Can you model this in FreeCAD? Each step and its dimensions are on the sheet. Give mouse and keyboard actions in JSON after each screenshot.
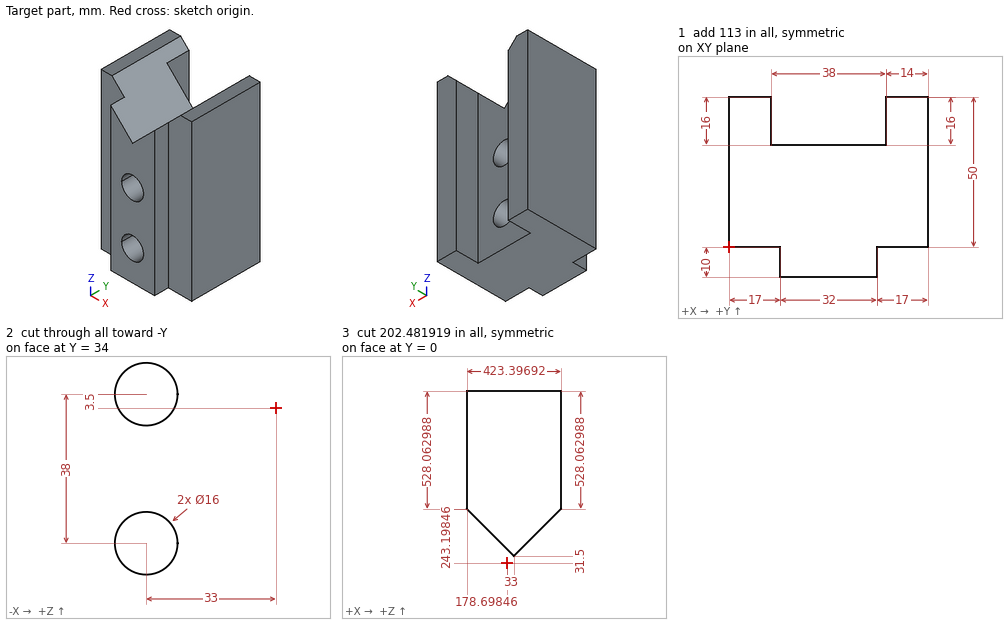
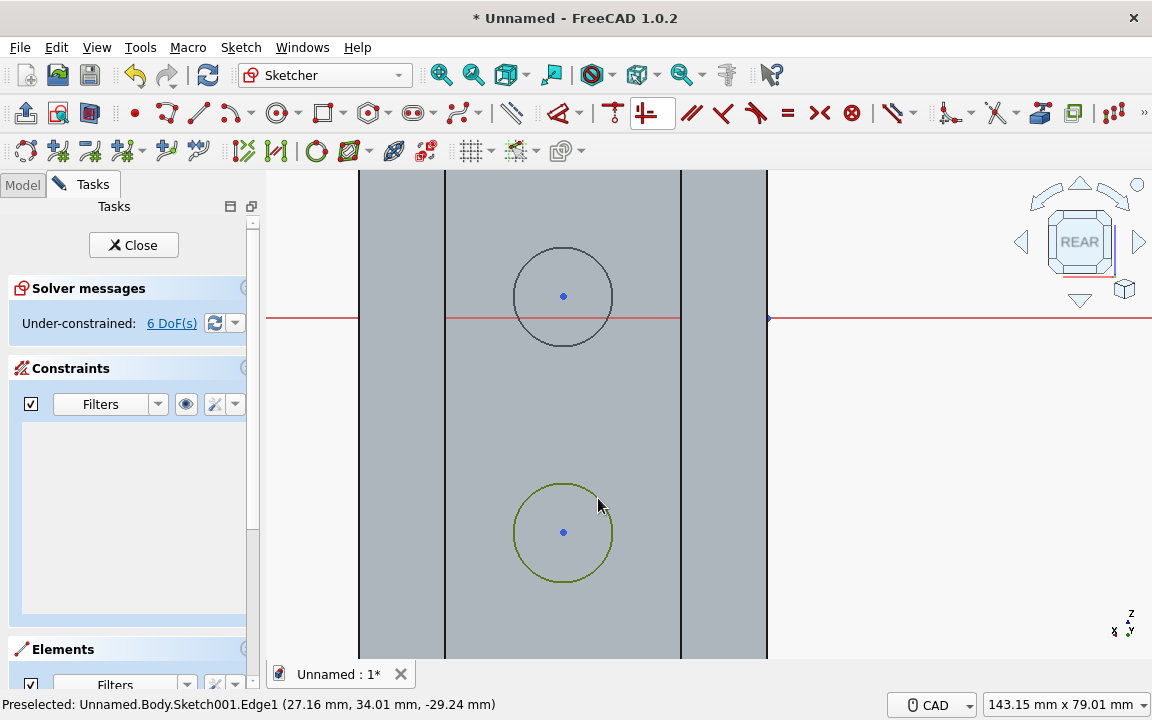
{"action": "left_click", "coordinate": [598, 262]}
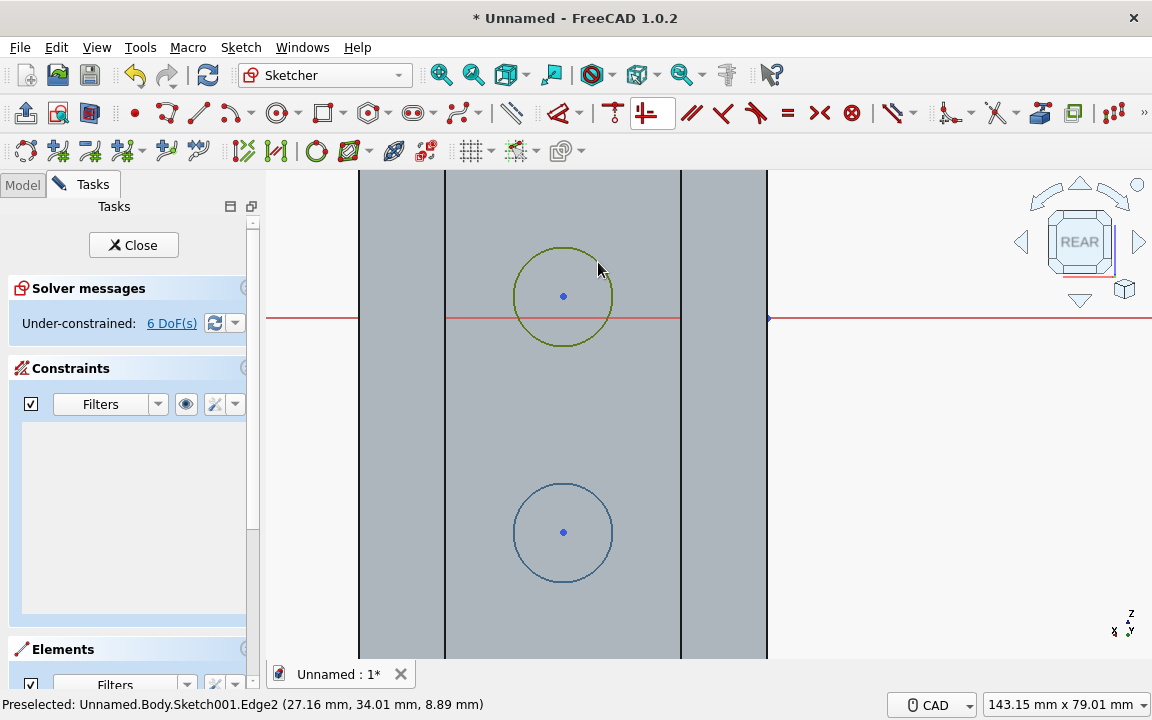
{"action": "left_click", "coordinate": [788, 114]}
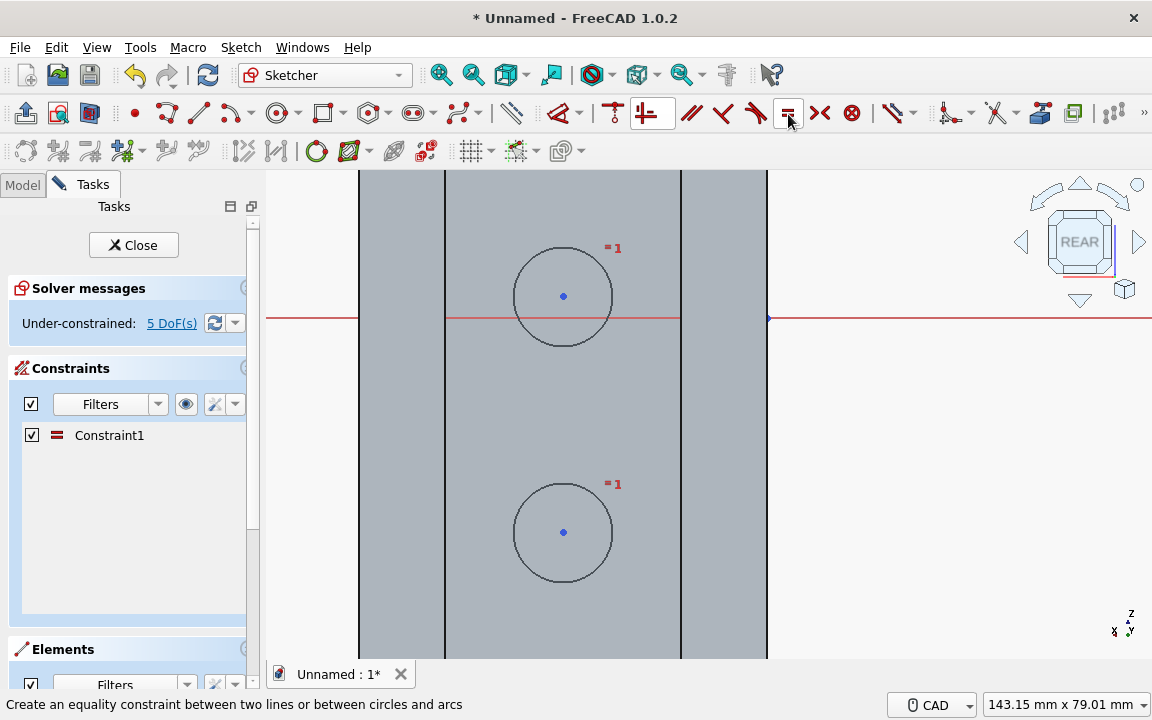
{"action": "left_click", "coordinate": [563, 533]}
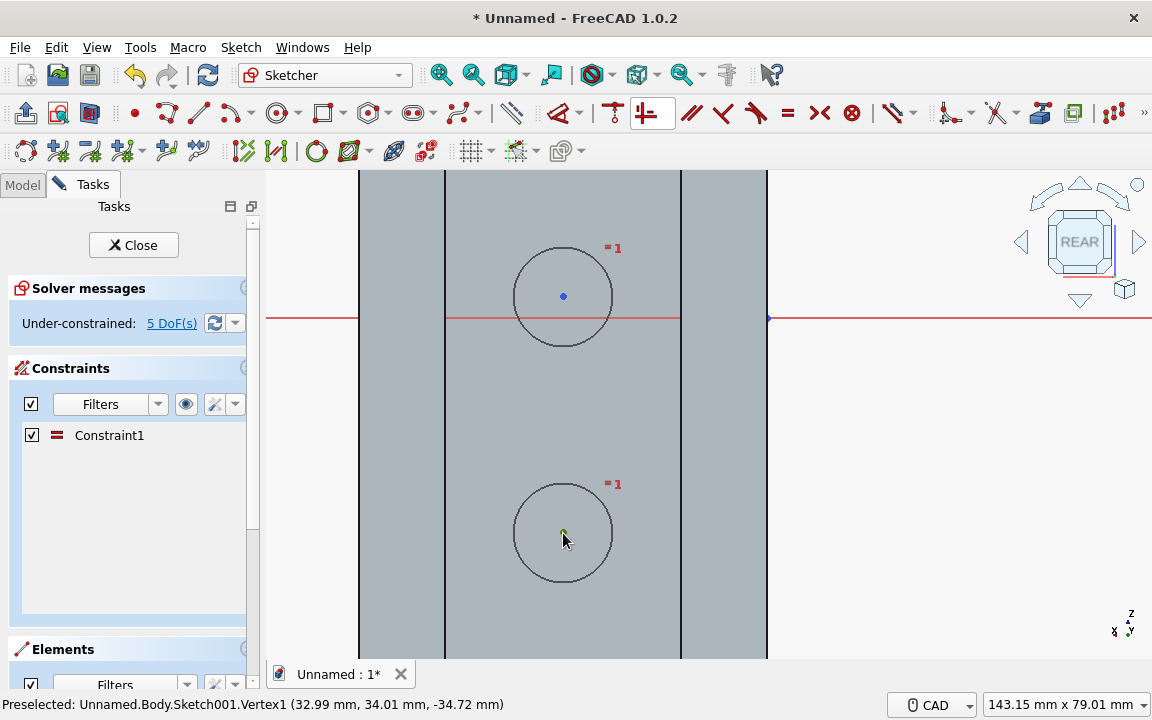
{"action": "left_click", "coordinate": [563, 297]}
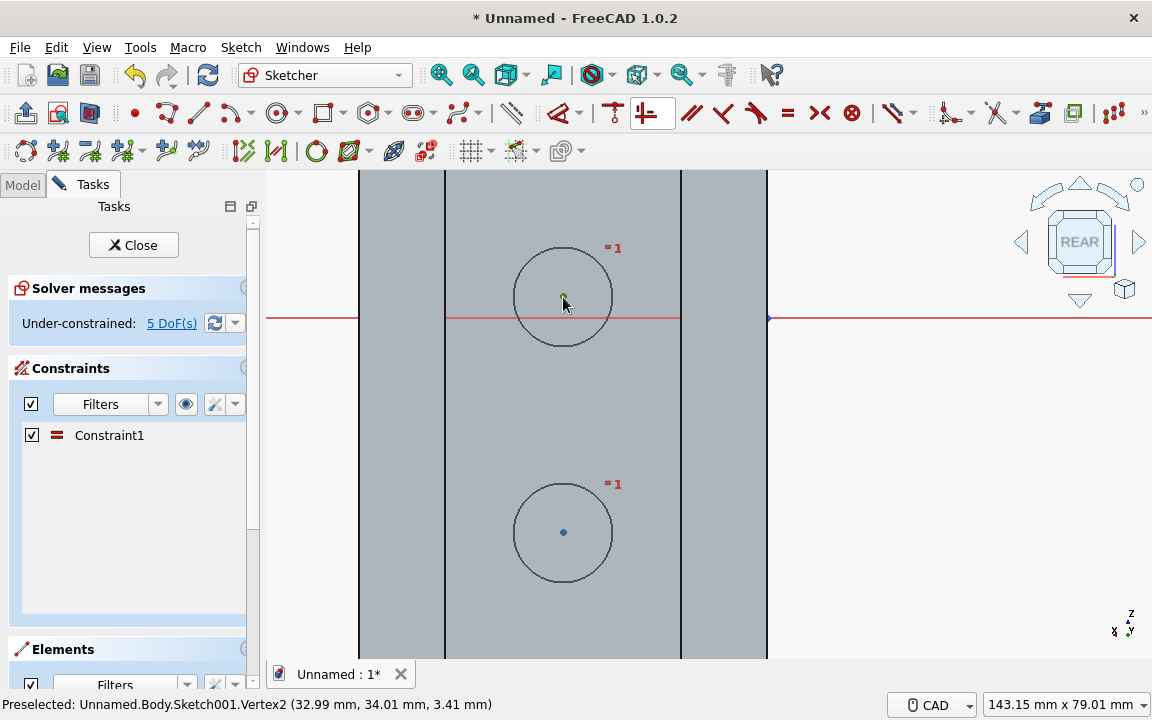
{"action": "key", "text": "v"}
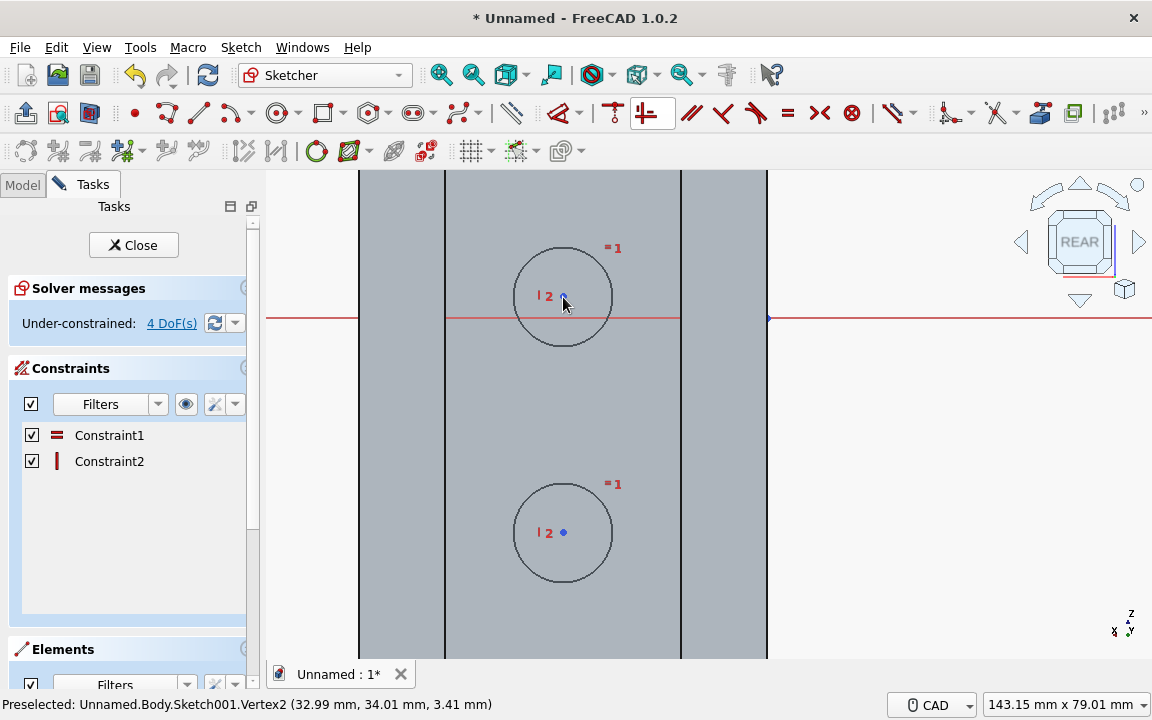
{"action": "left_click", "coordinate": [558, 114]}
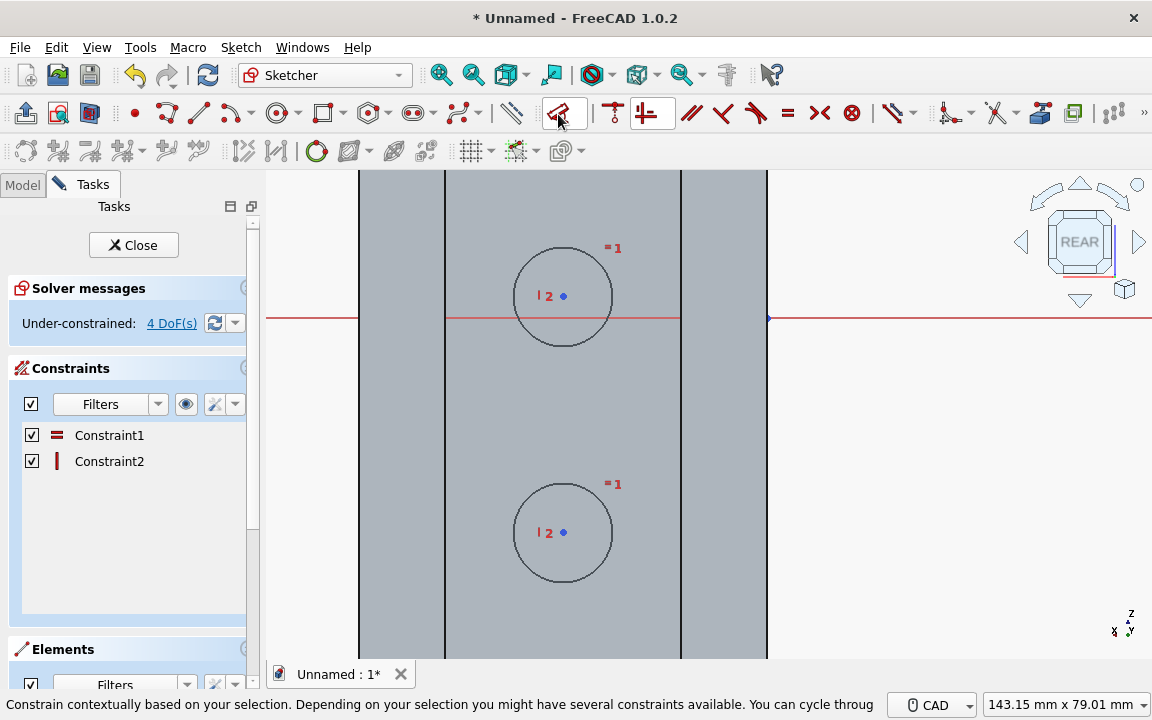
{"action": "left_click", "coordinate": [598, 498]}
{"action": "left_click", "coordinate": [621, 475]}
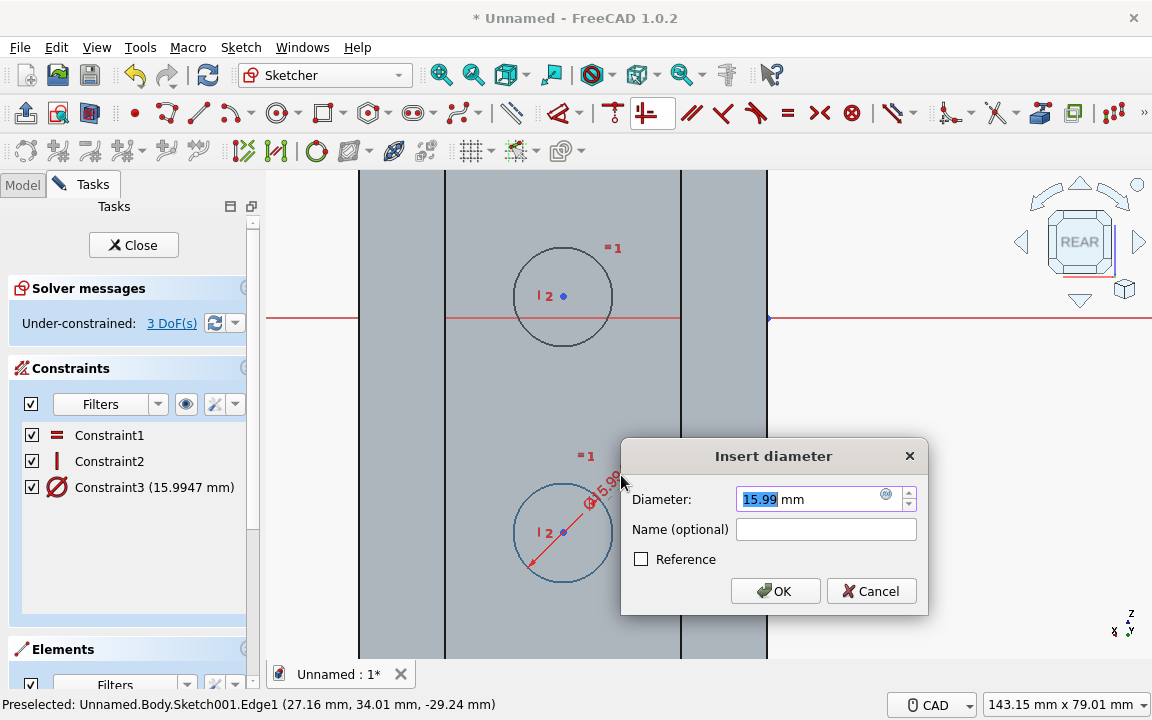
{"action": "type", "text": "16"}
{"action": "key", "text": "Return"}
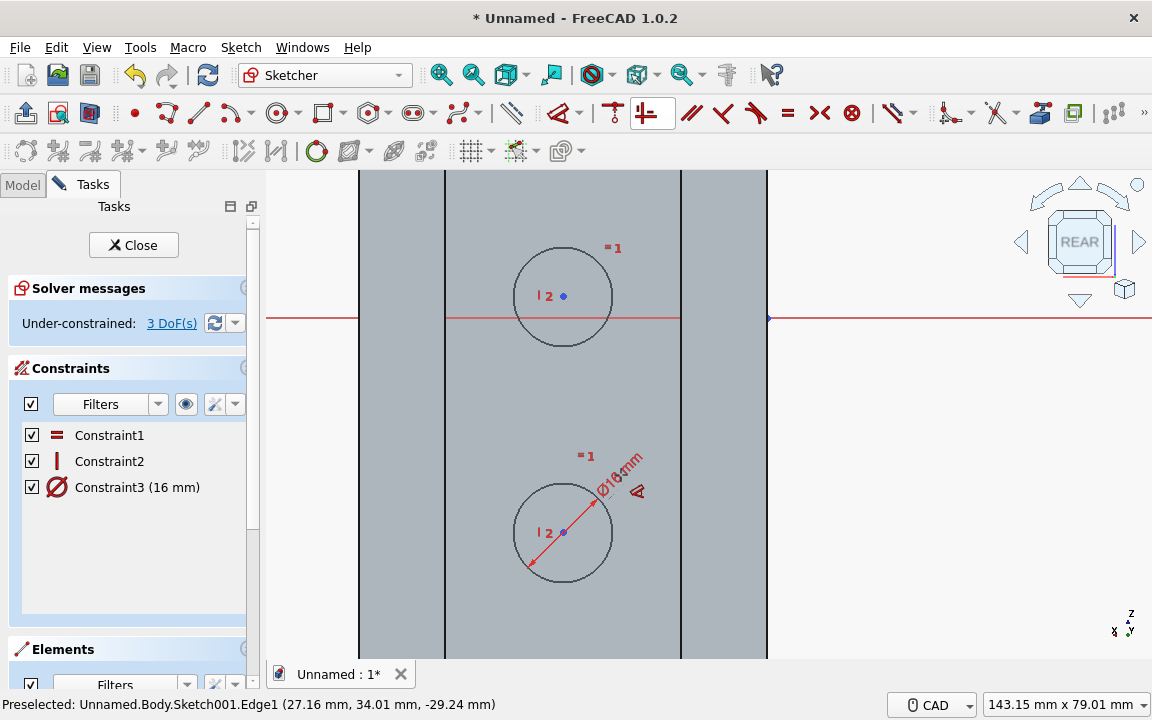
{"action": "left_click", "coordinate": [563, 533]}
{"action": "left_click", "coordinate": [665, 567]}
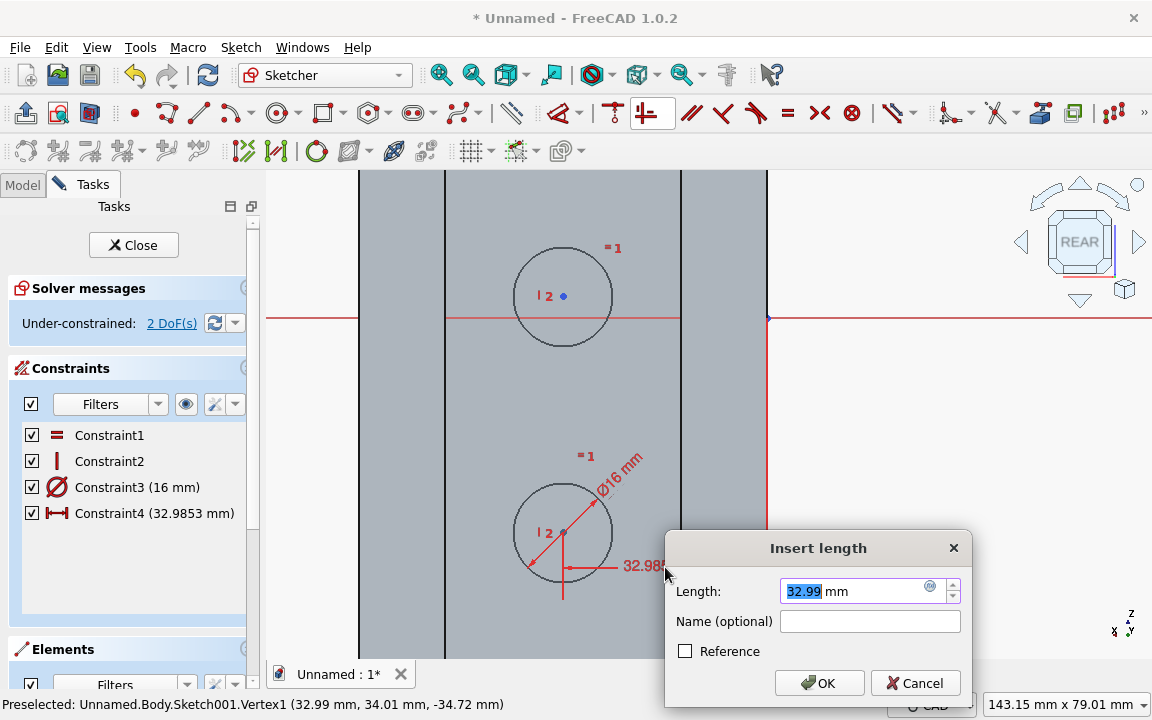
{"action": "type", "text": "33"}
{"action": "key", "text": "Return"}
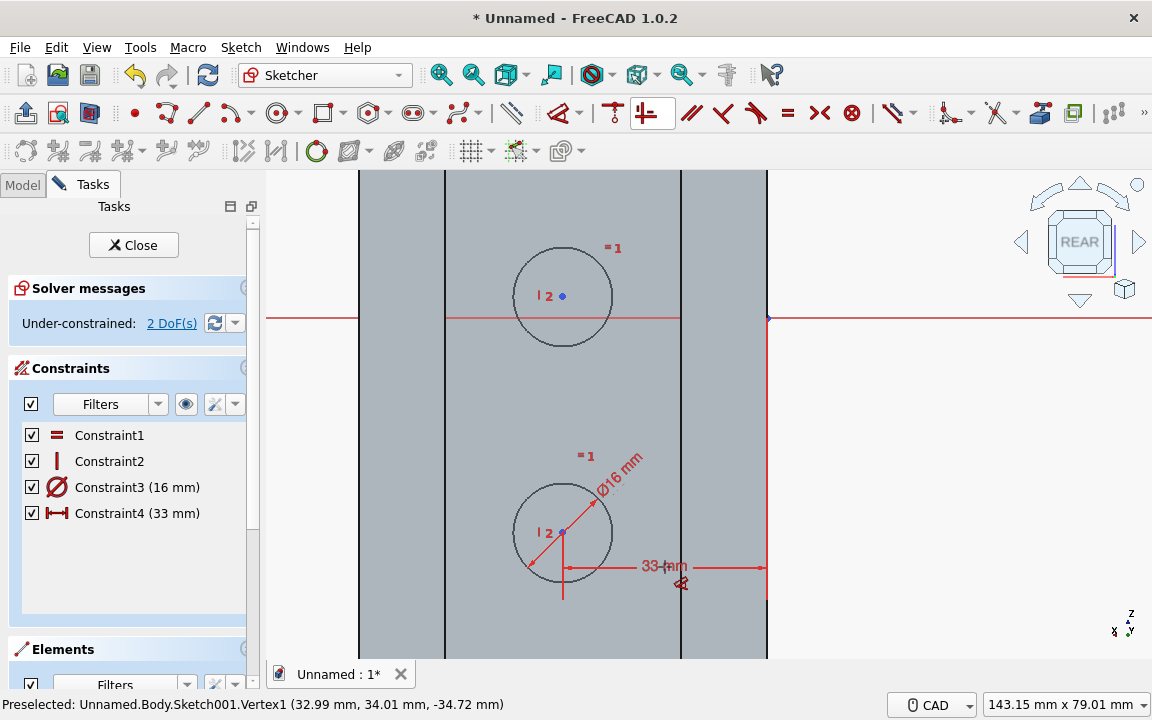
{"action": "scroll", "coordinate": [563, 297], "scroll_direction": "up", "scroll_amount": 4}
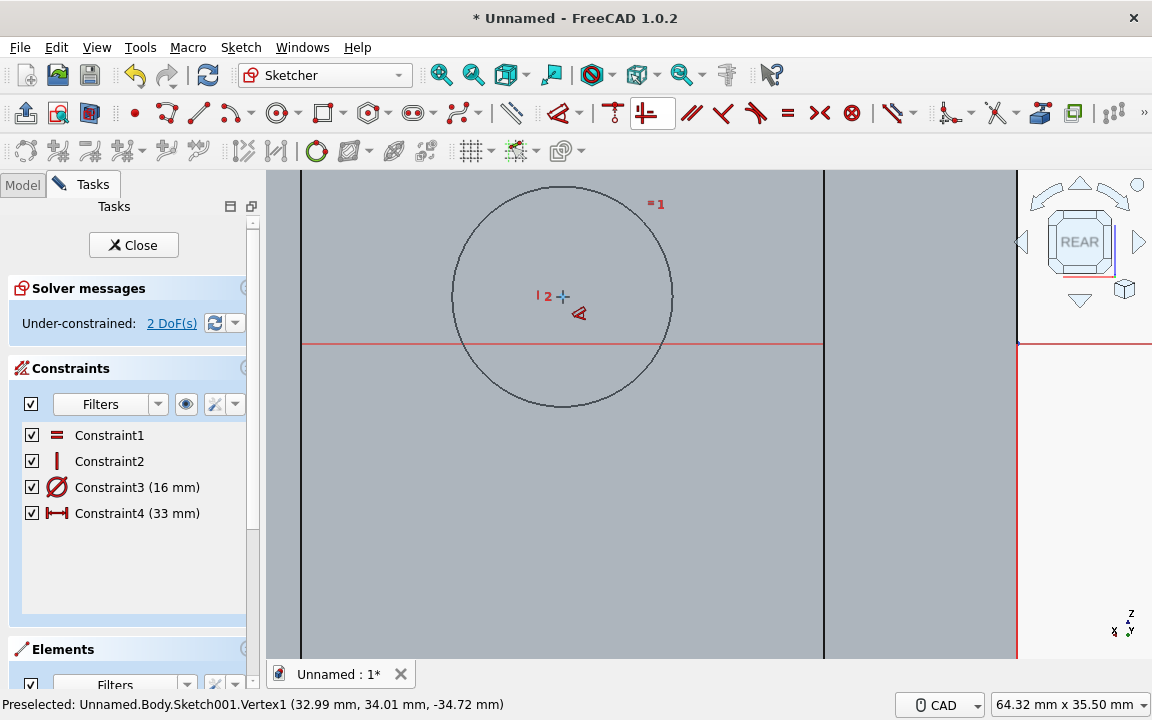
{"action": "left_click", "coordinate": [562, 297]}
{"action": "left_click", "coordinate": [528, 320]}